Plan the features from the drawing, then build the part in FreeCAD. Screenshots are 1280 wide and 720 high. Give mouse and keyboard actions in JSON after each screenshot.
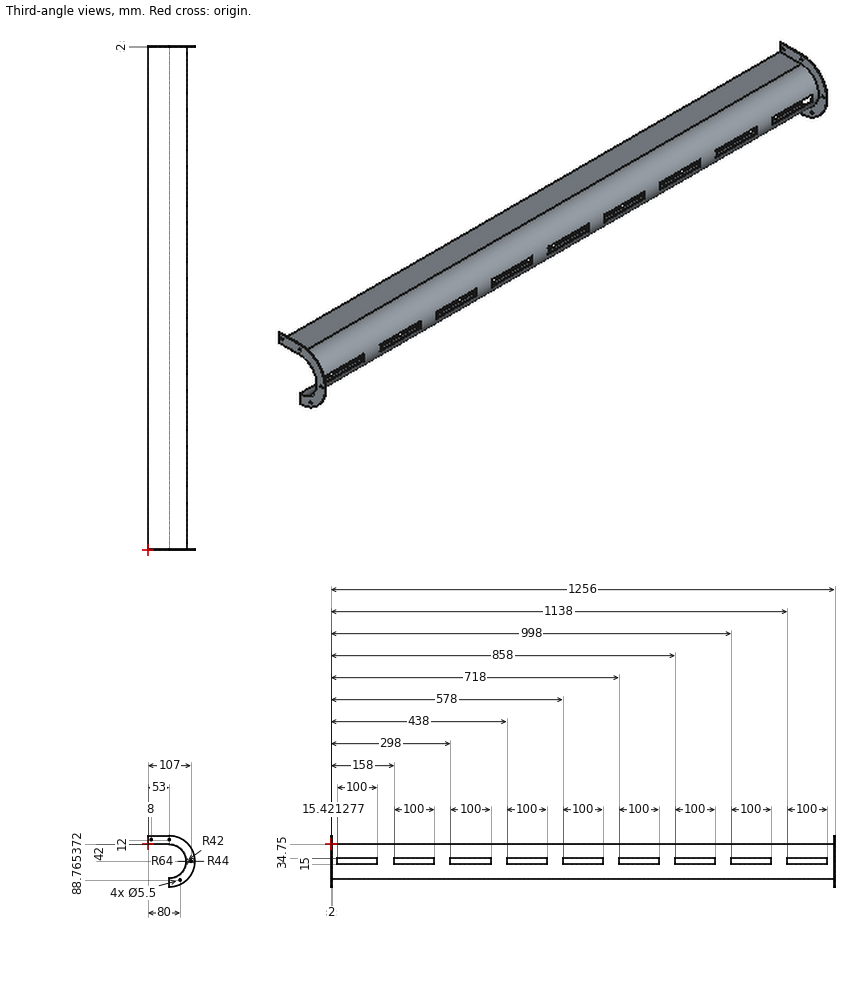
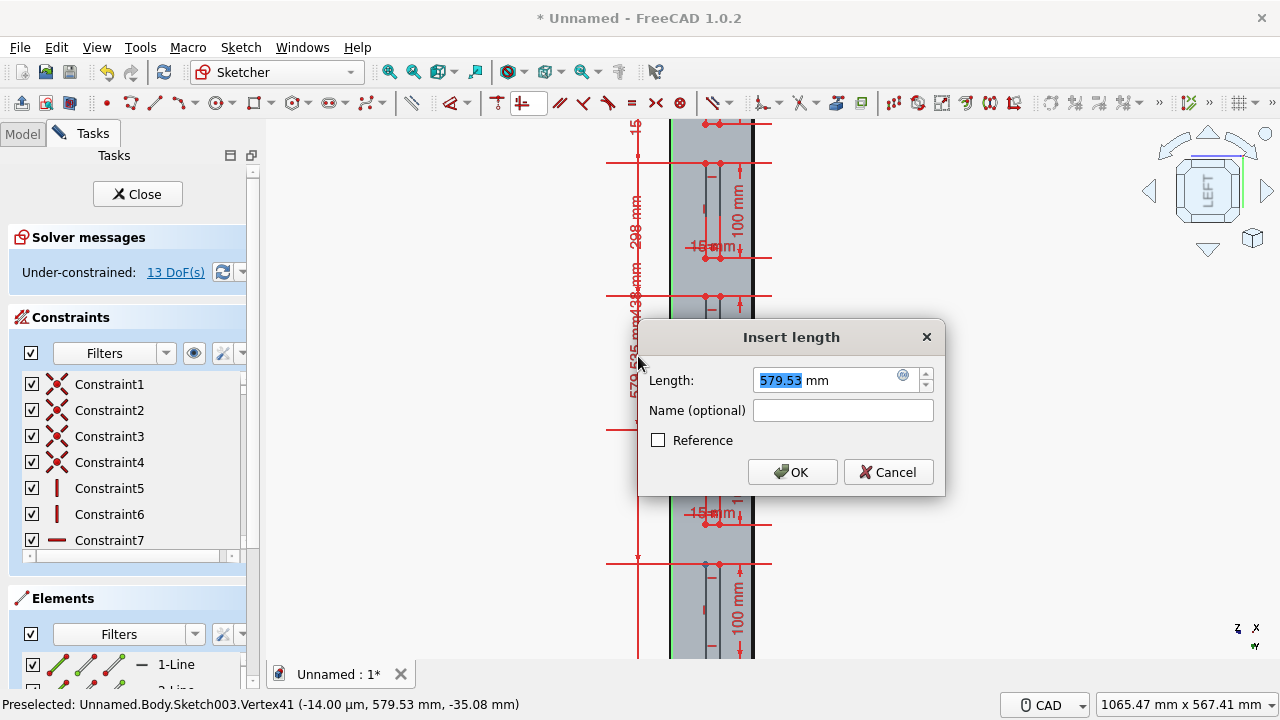
{"action": "type", "text": "578"}
{"action": "key", "text": "Return"}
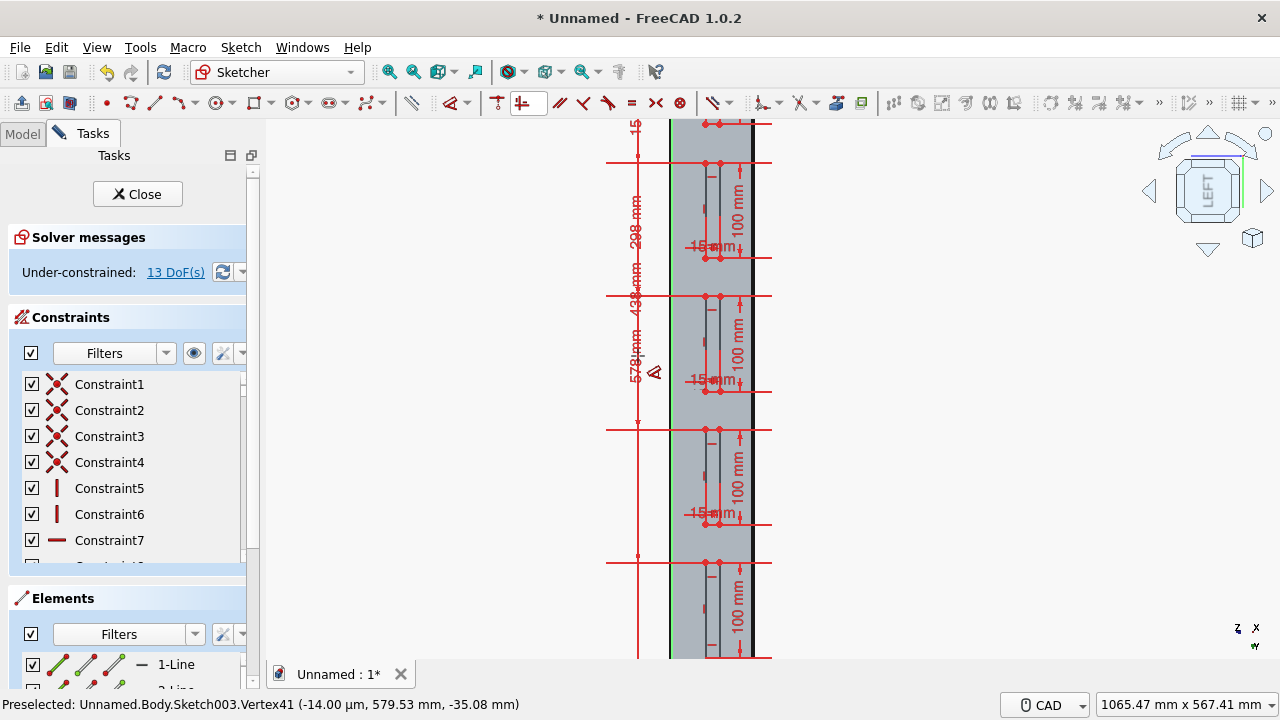
{"action": "scroll", "coordinate": [708, 297], "scroll_direction": "down", "scroll_amount": 6}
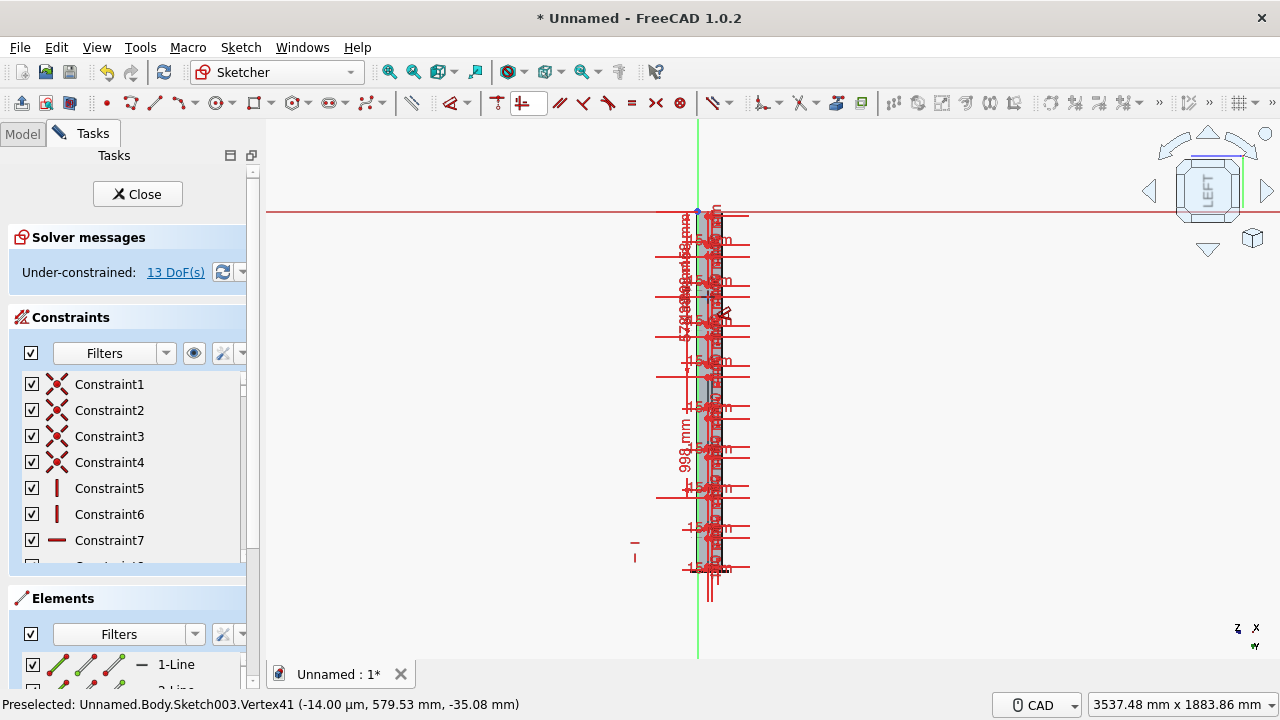
{"action": "scroll", "coordinate": [708, 419], "scroll_direction": "up", "scroll_amount": 6}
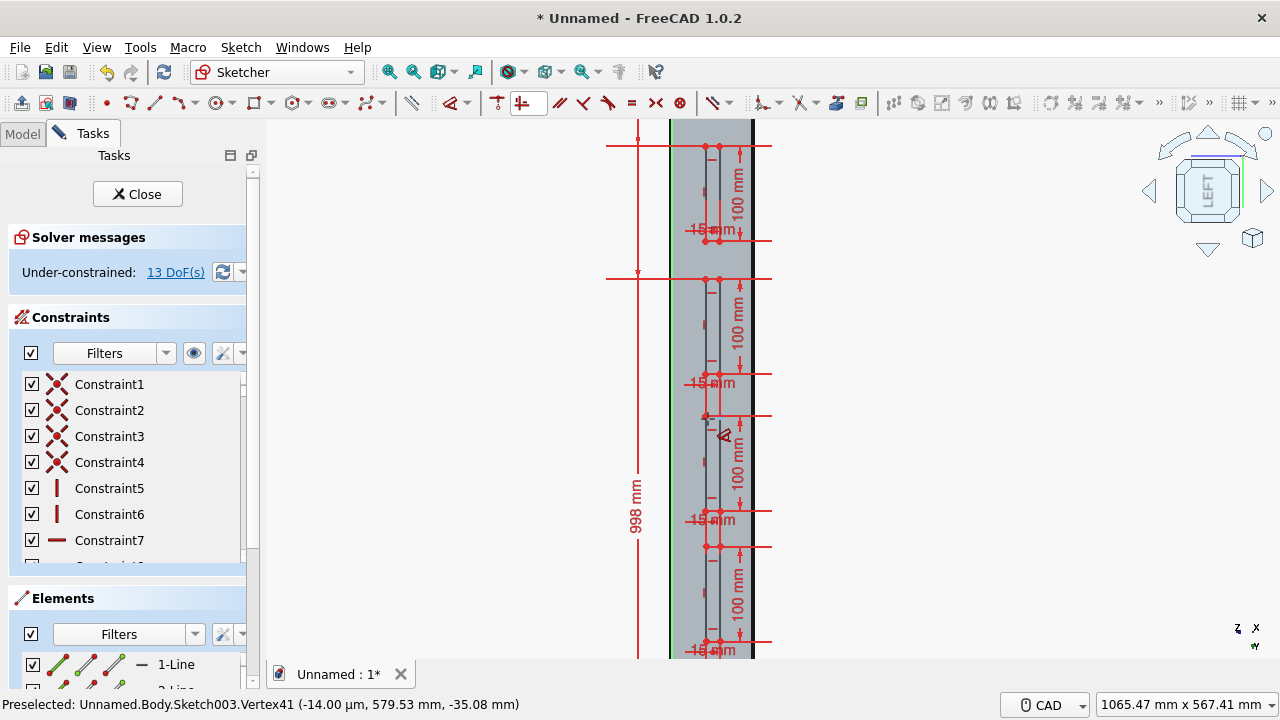
{"action": "left_click", "coordinate": [706, 416]}
{"action": "left_click", "coordinate": [638, 282]}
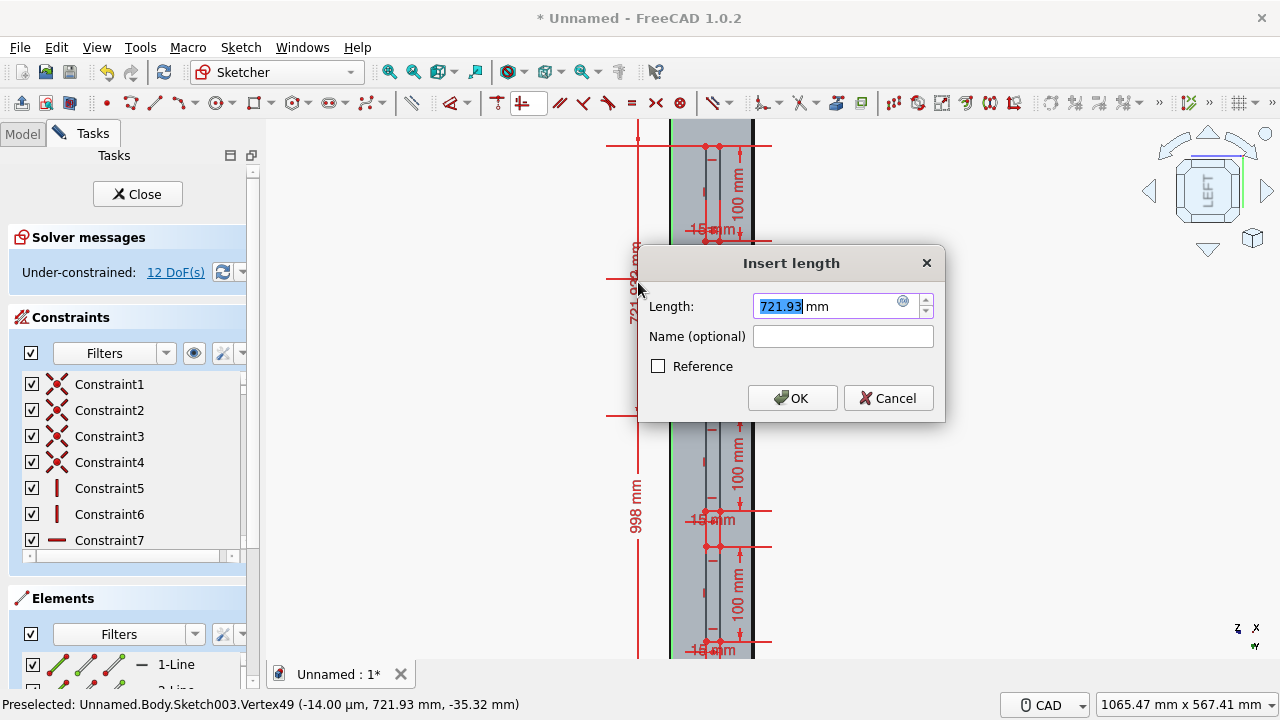
{"action": "type", "text": "718"}
{"action": "key", "text": "Return"}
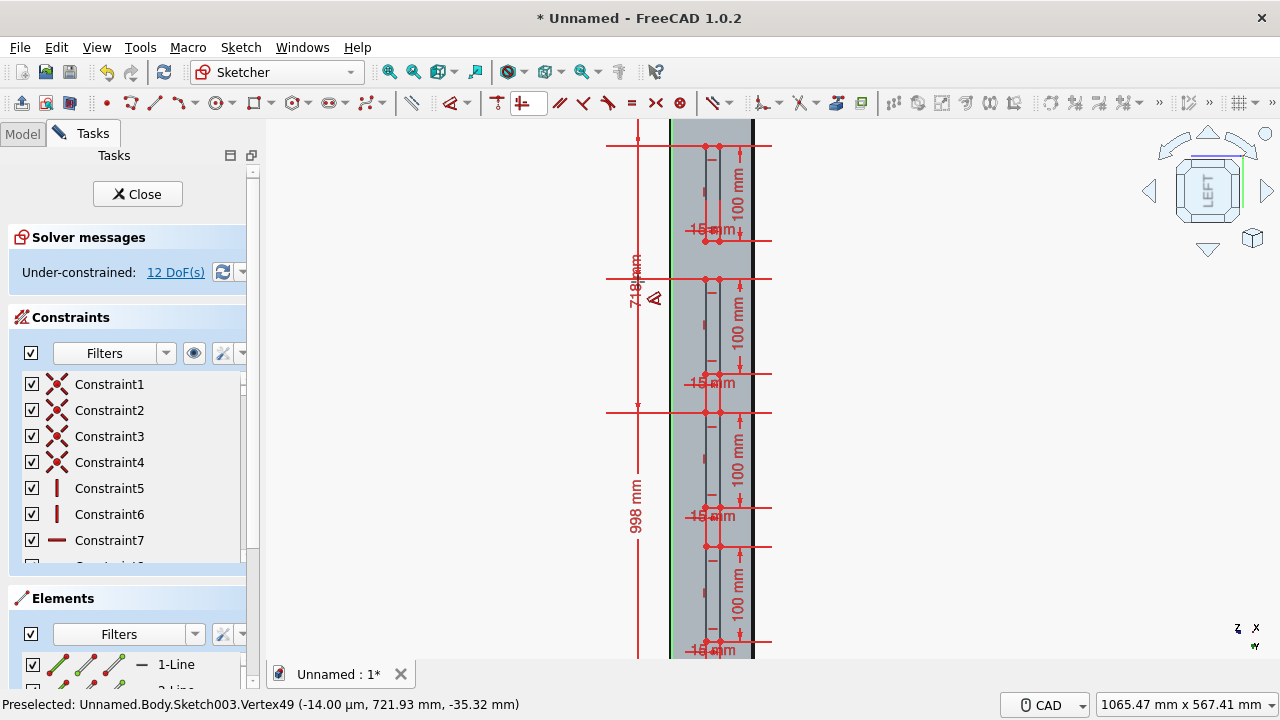
{"action": "left_click", "coordinate": [706, 547]}
{"action": "left_click", "coordinate": [638, 347]}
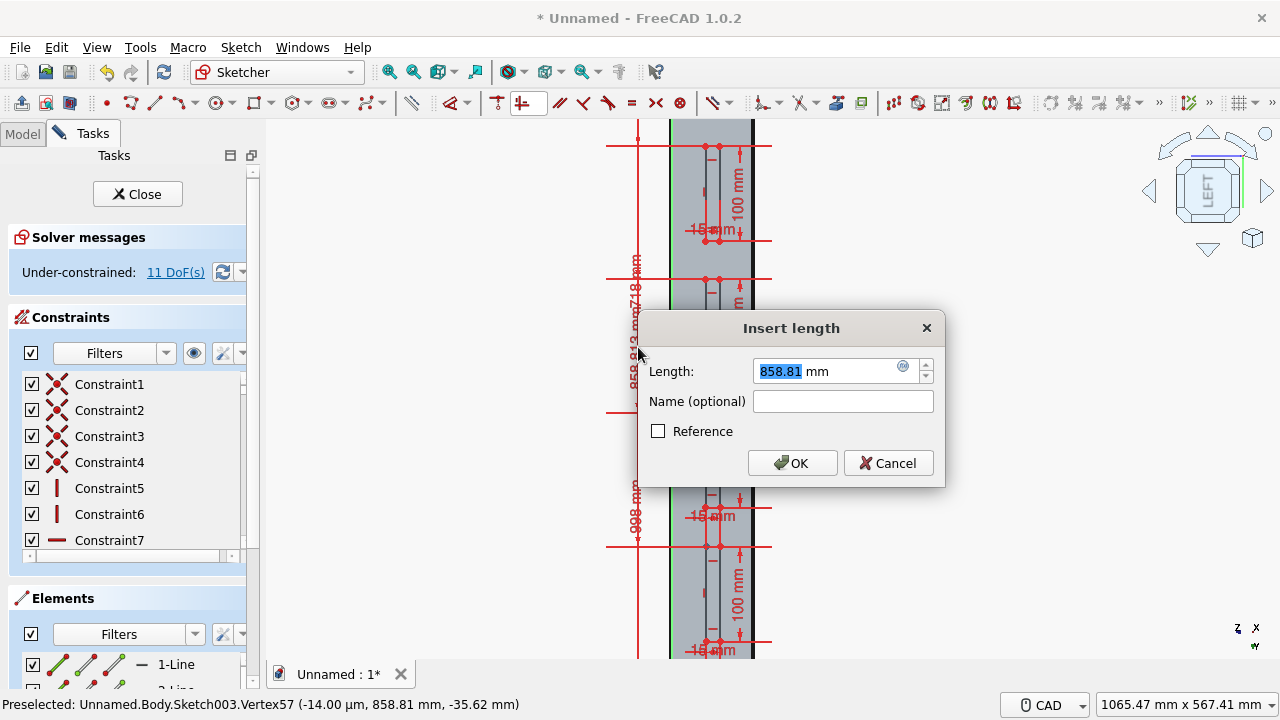
{"action": "type", "text": "858"}
{"action": "key", "text": "Return"}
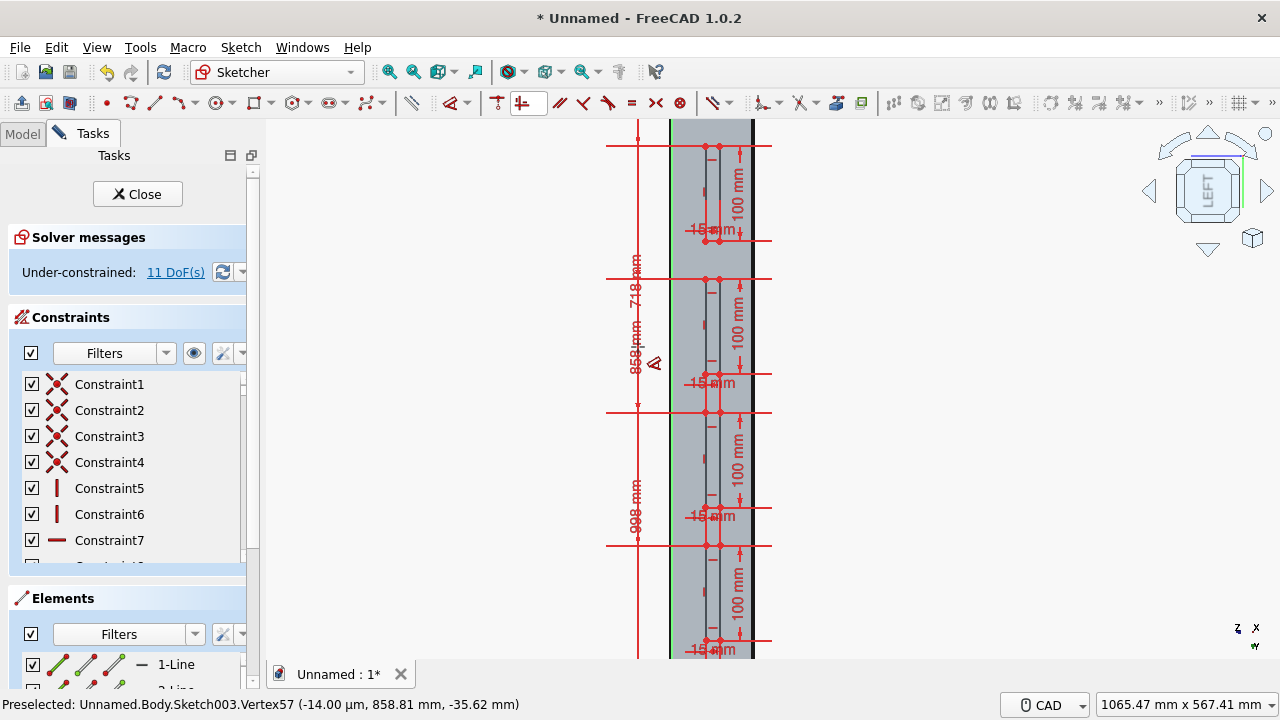
{"action": "scroll", "coordinate": [708, 419], "scroll_direction": "down", "scroll_amount": 6}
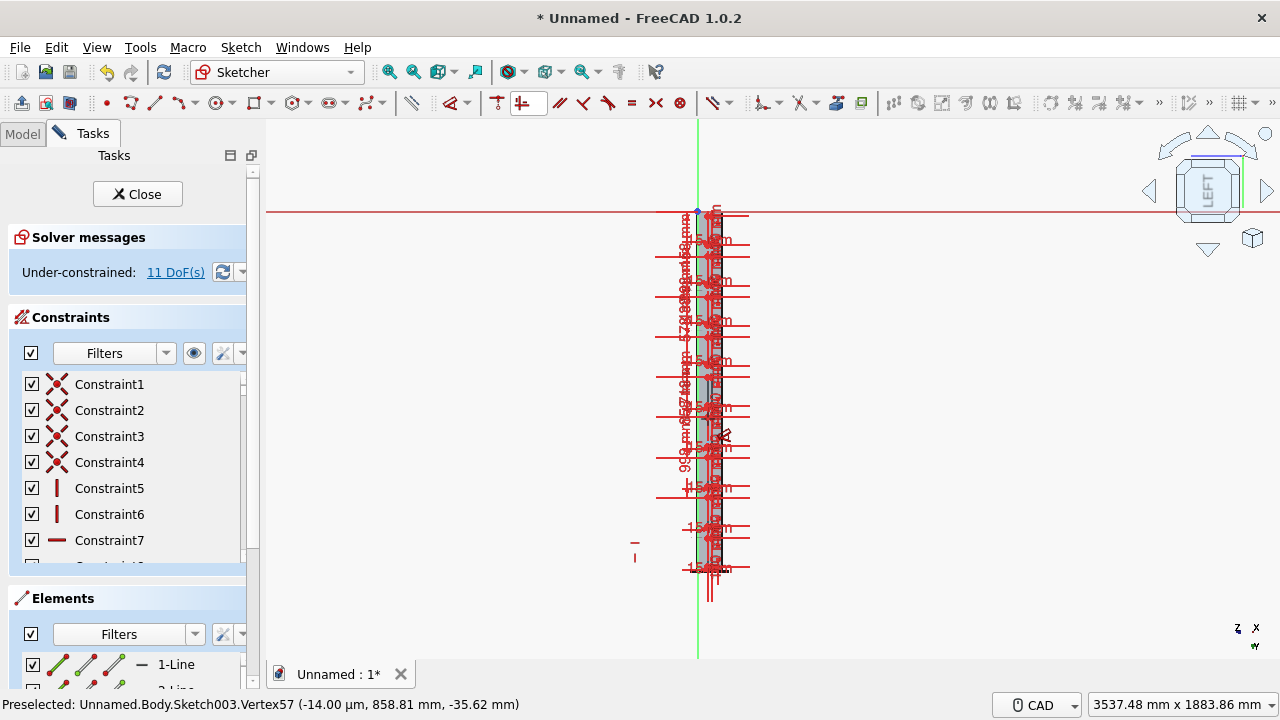
{"action": "scroll", "coordinate": [708, 538], "scroll_direction": "up", "scroll_amount": 6}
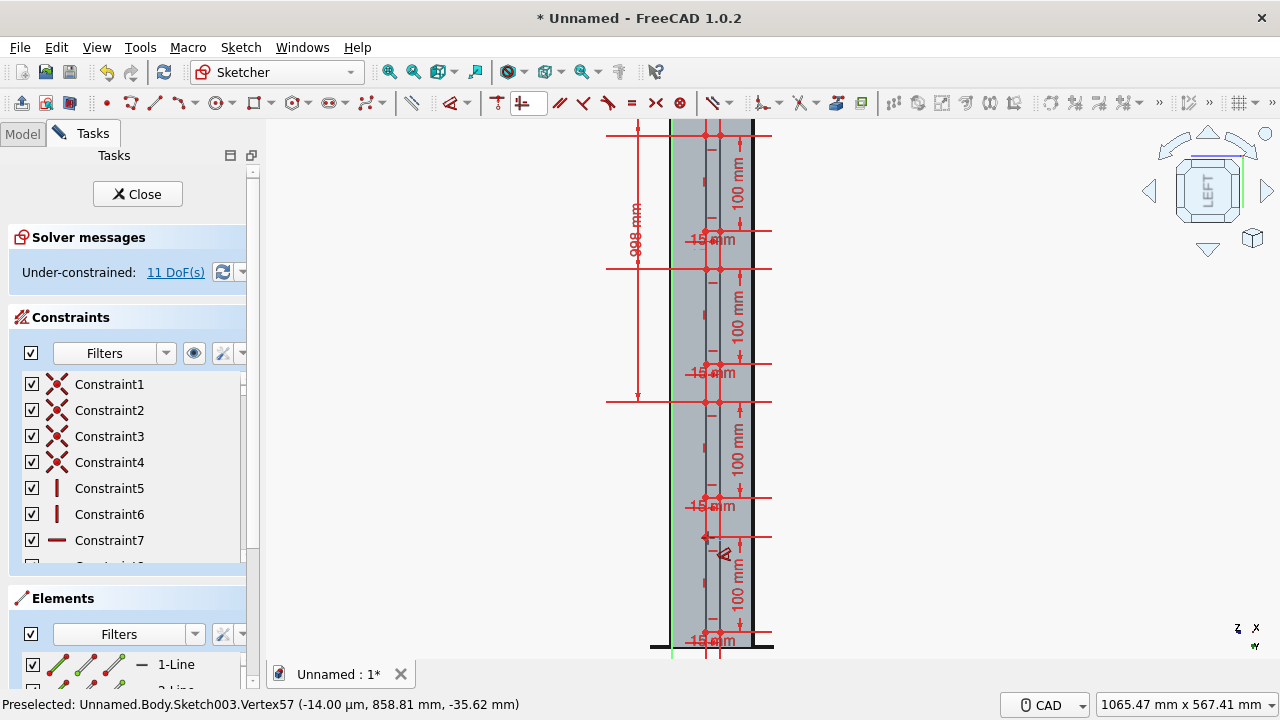
{"action": "left_click", "coordinate": [706, 537]}
{"action": "left_click", "coordinate": [638, 342]}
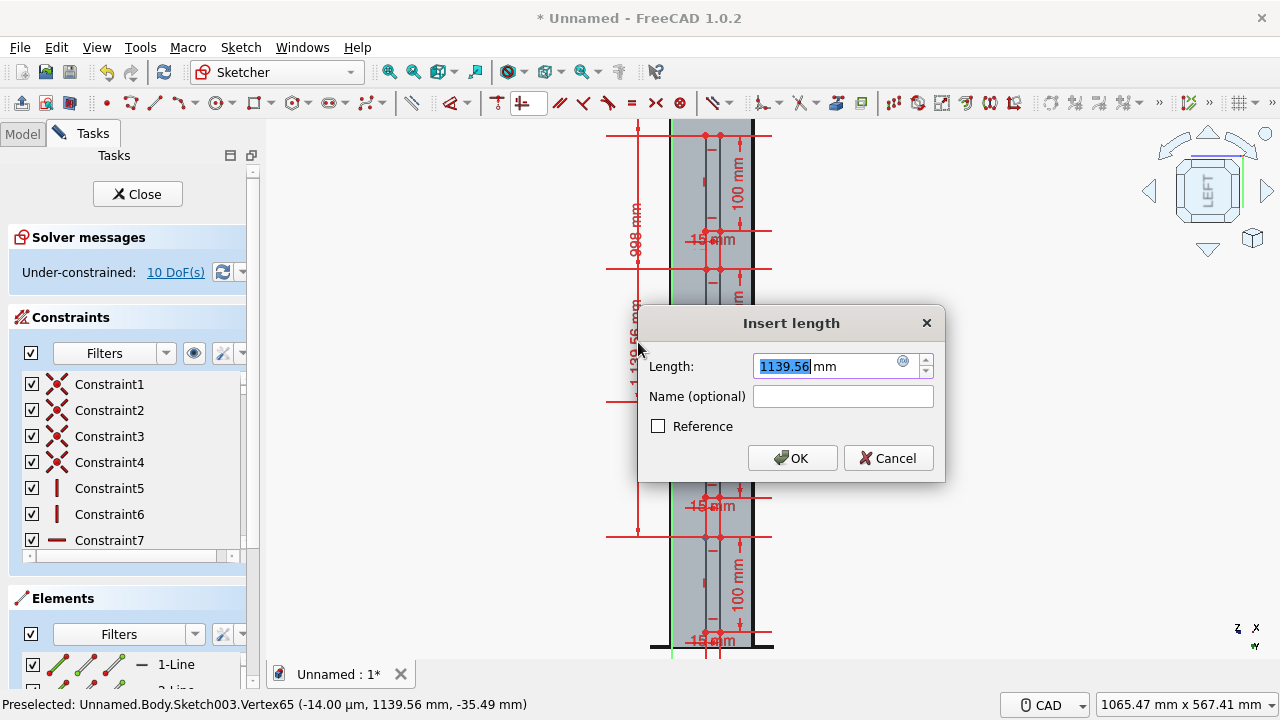
{"action": "type", "text": "1138"}
{"action": "key", "text": "Return"}